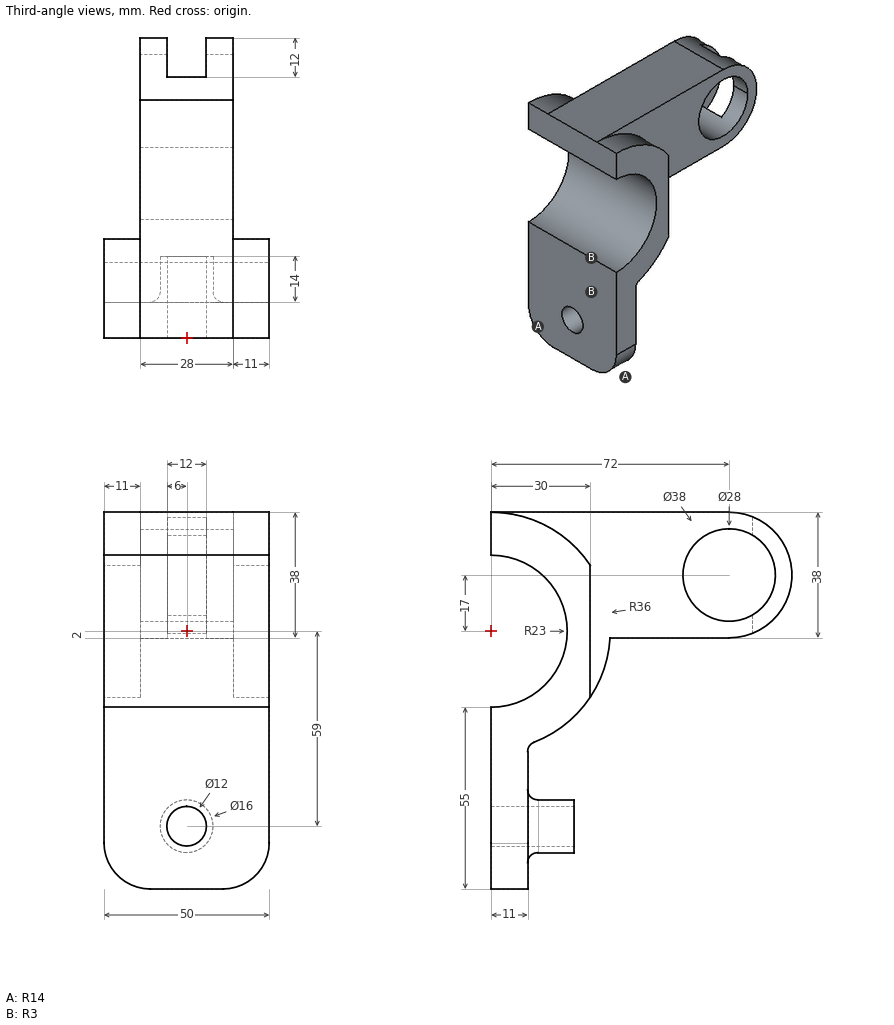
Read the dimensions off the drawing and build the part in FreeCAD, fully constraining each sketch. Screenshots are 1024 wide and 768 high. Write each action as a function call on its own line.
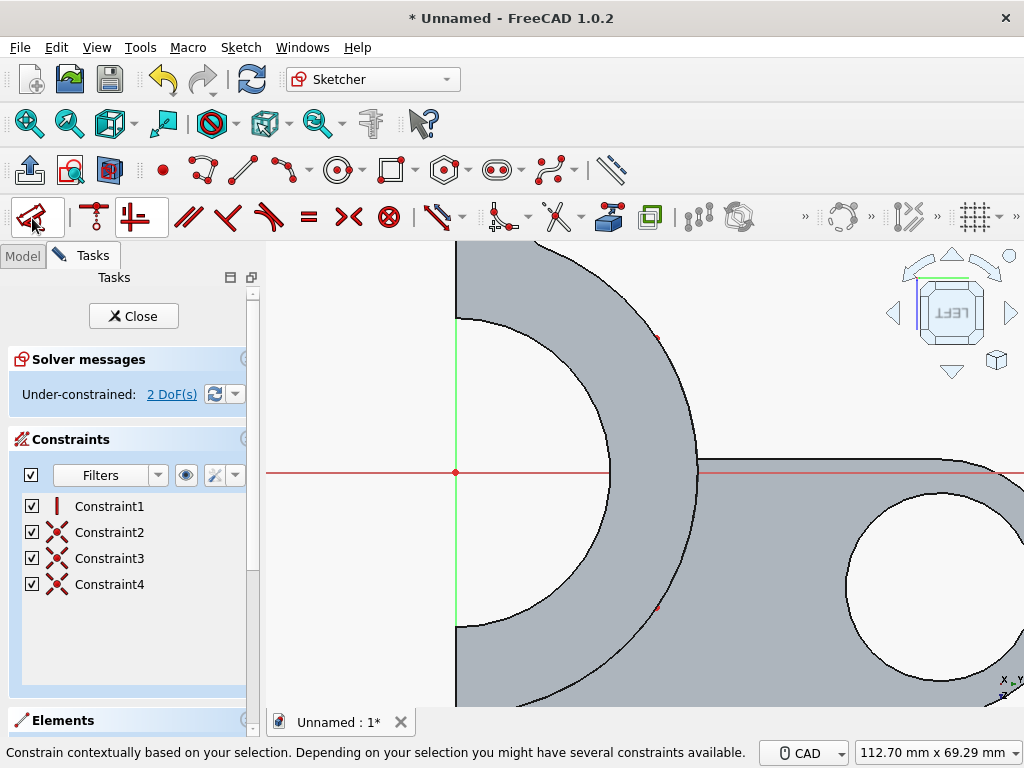
click(691, 529)
click(722, 536)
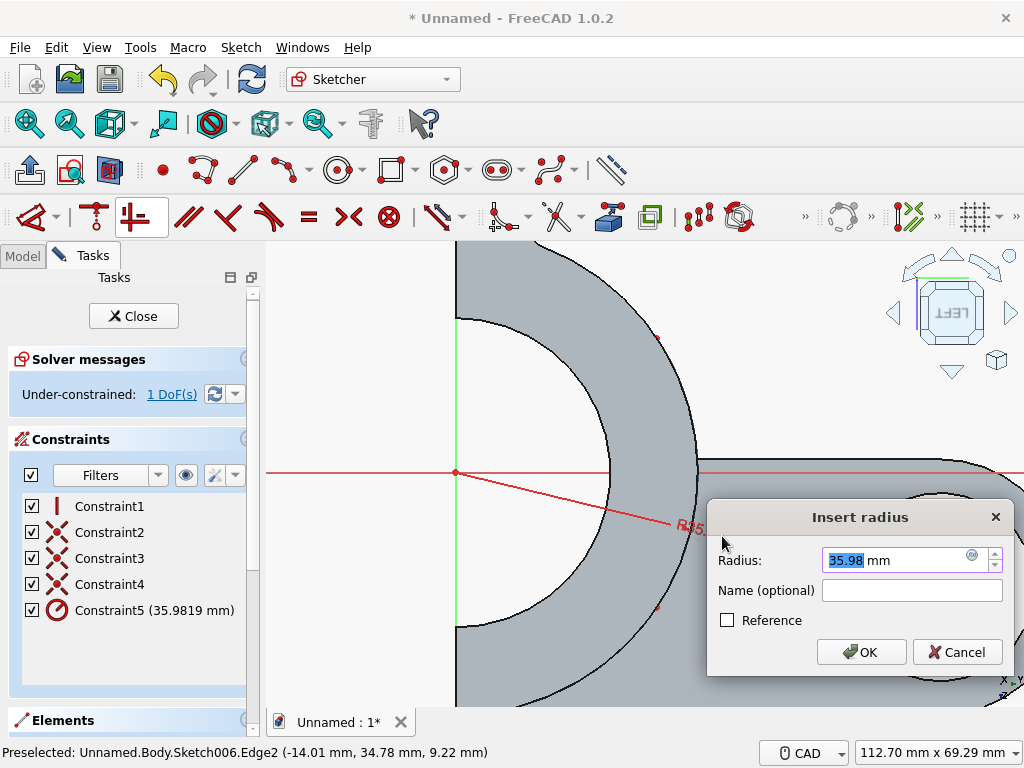
text(36)
key(Return)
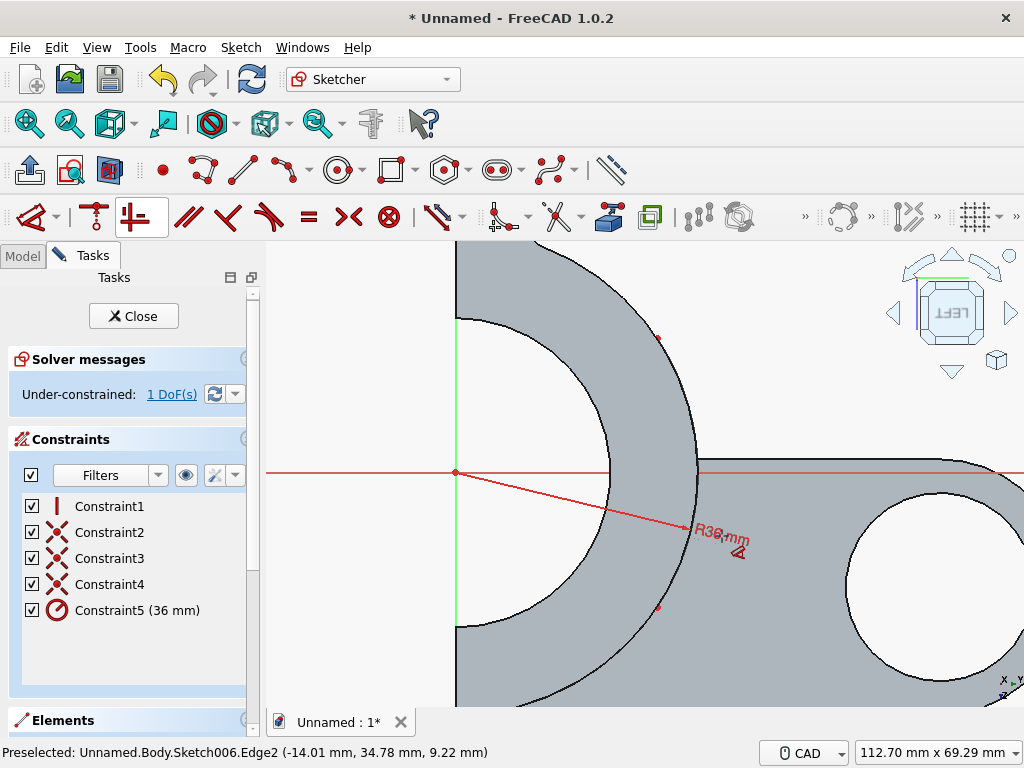
click(657, 338)
click(556, 304)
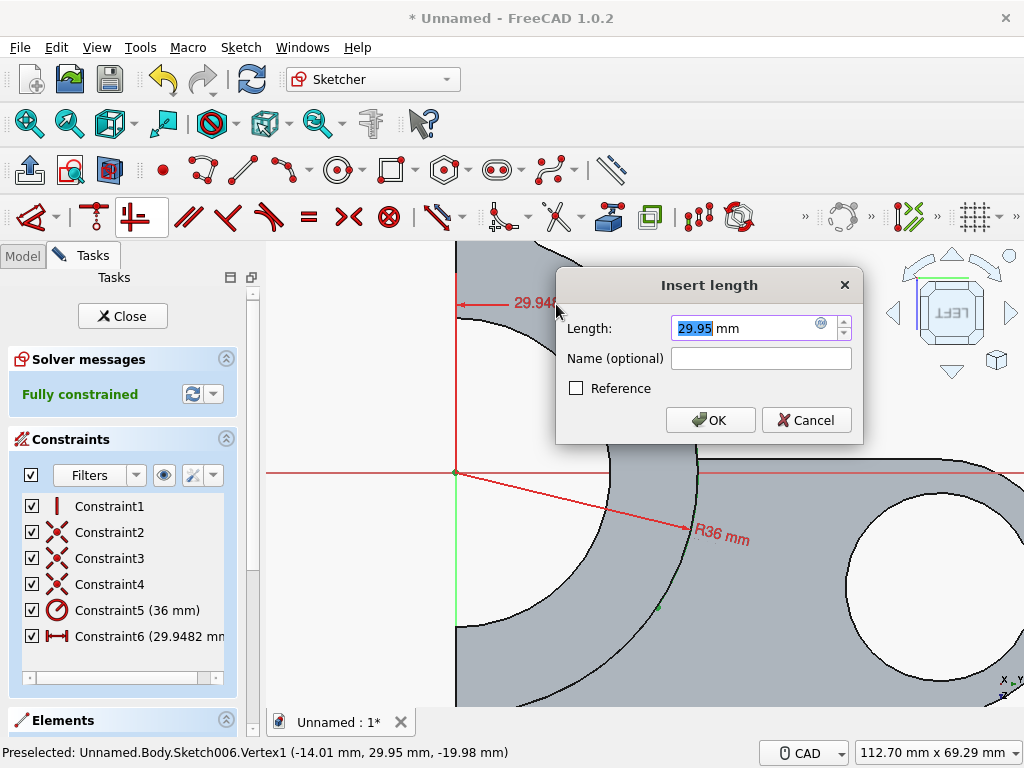
text(30)
key(Return)
key(Escape)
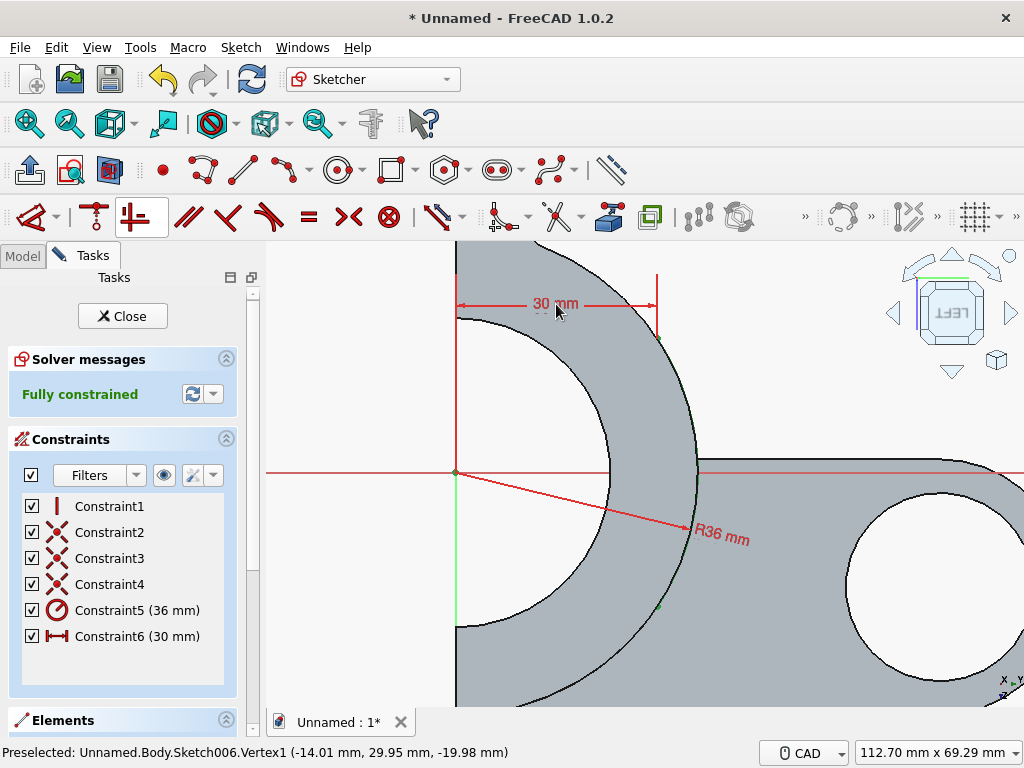
click(123, 316)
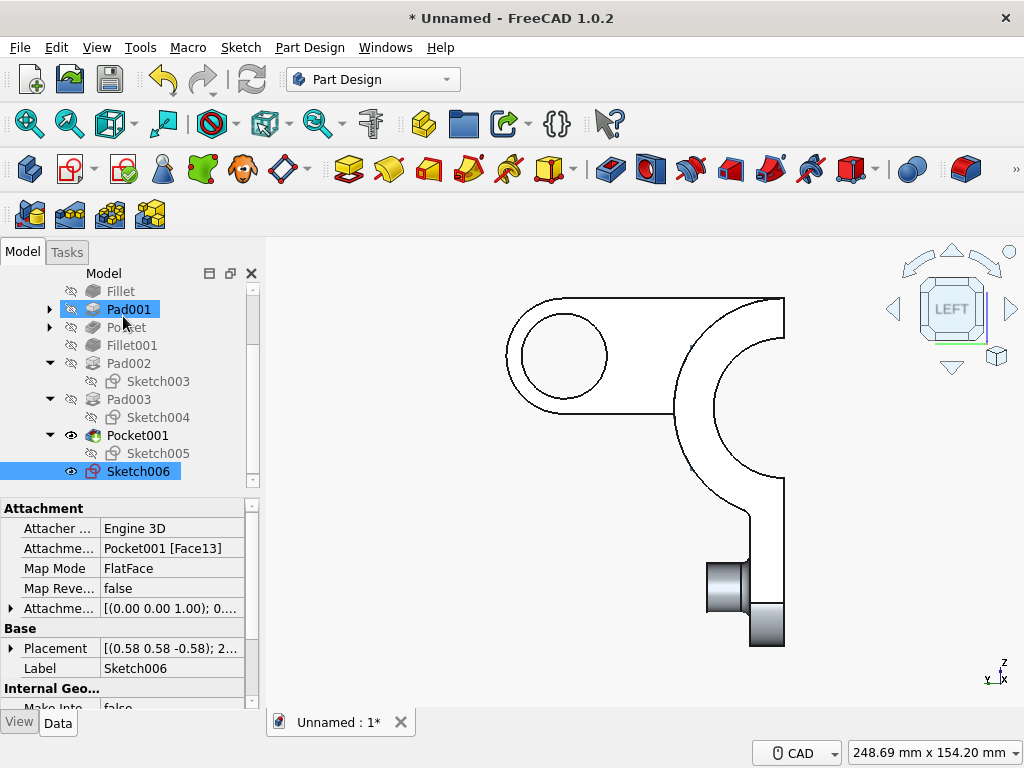
click(612, 170)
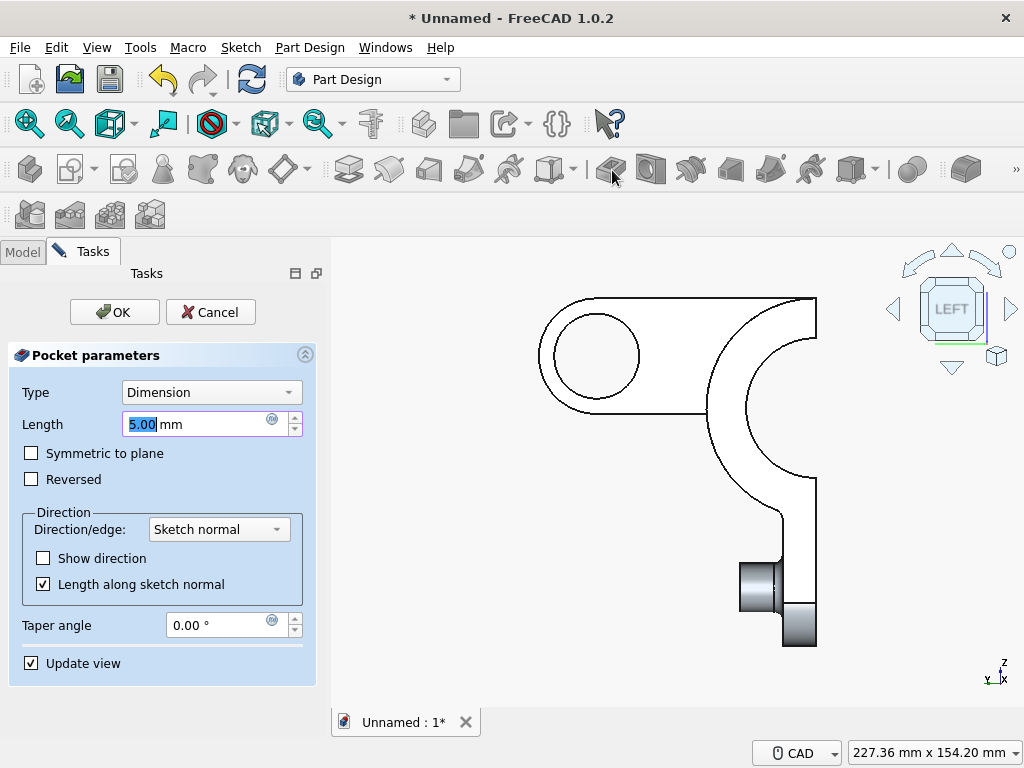
text(11)
key(Tab)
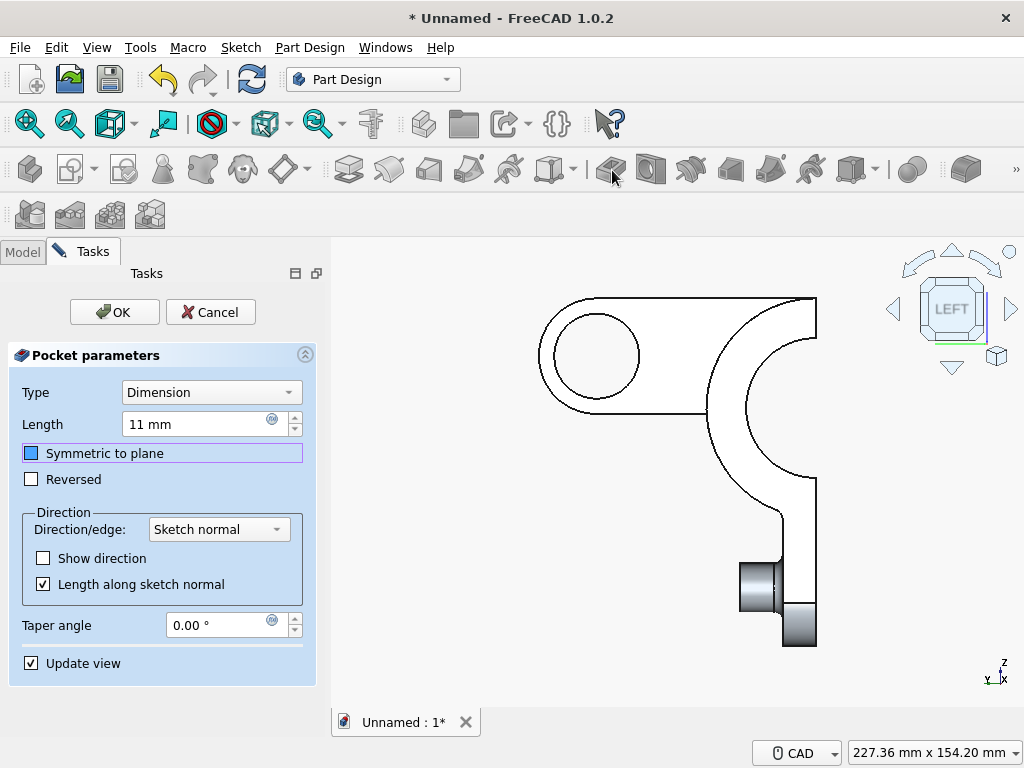
click(30, 479)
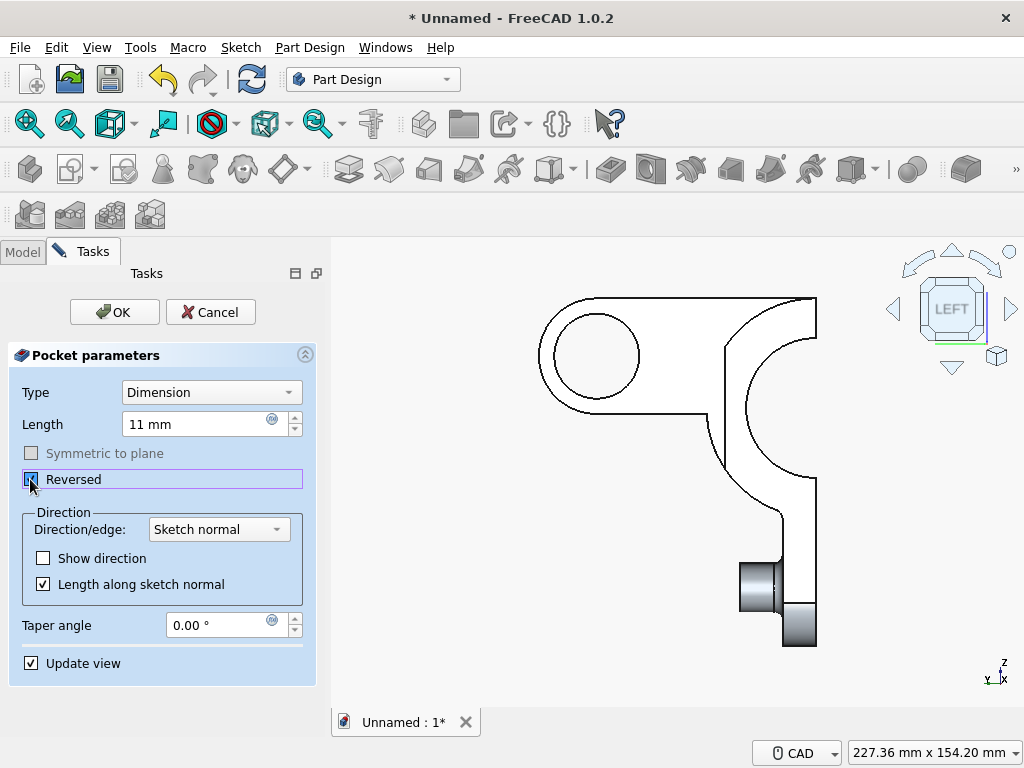
click(115, 312)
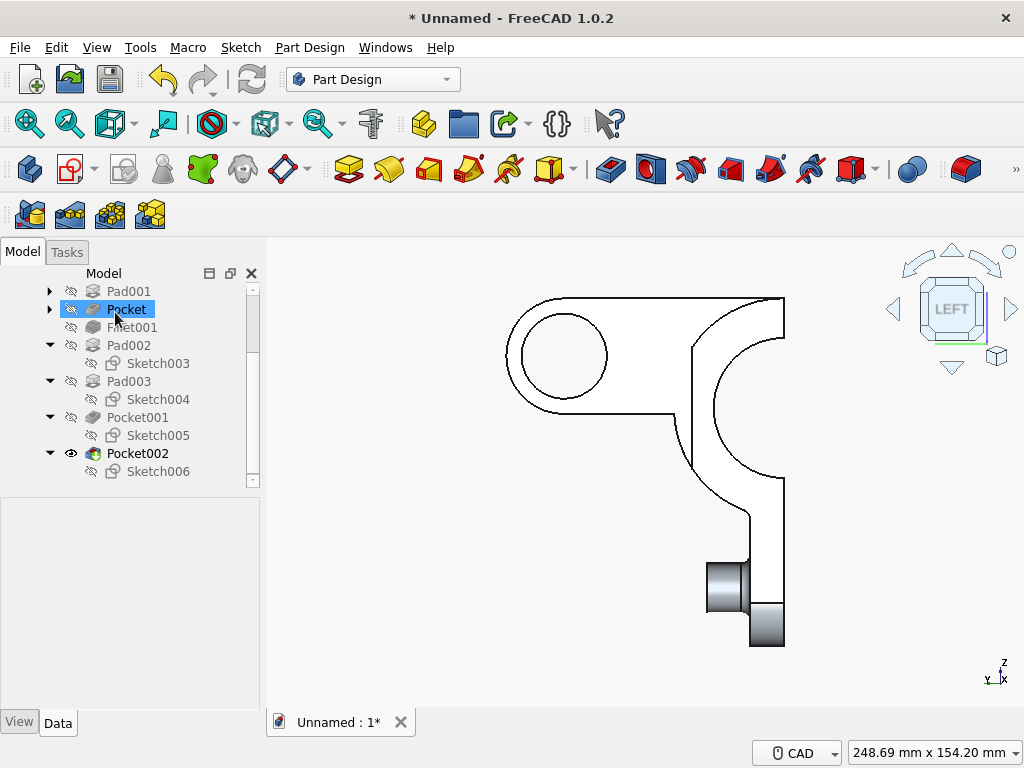
key(0)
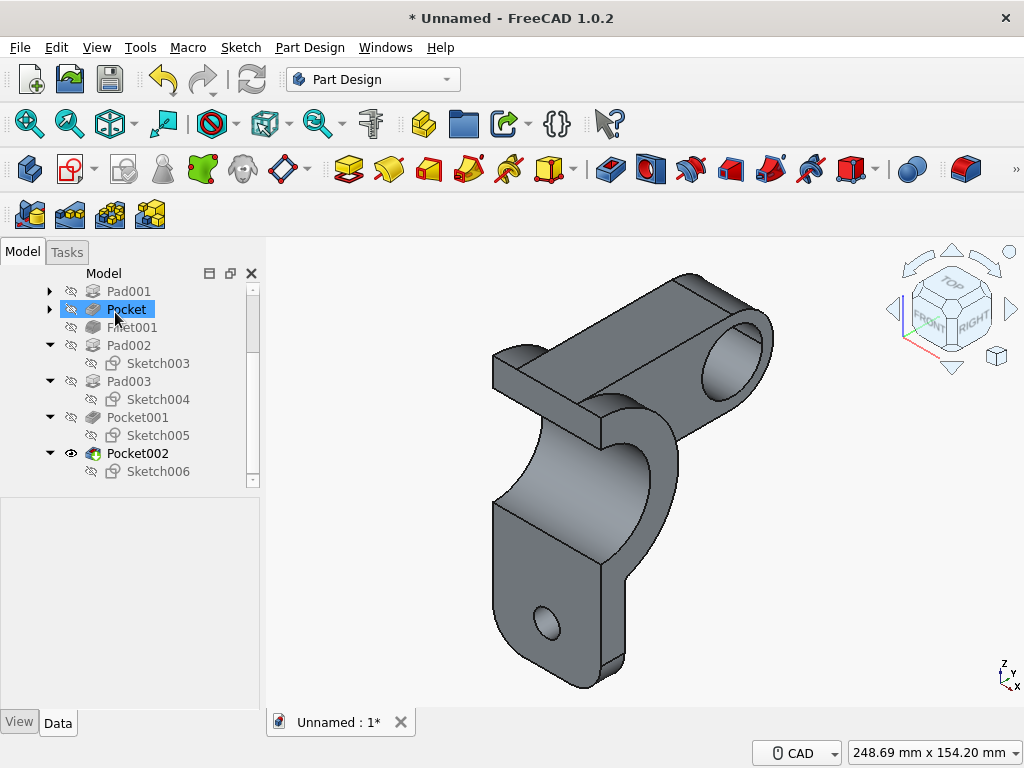
click(617, 567)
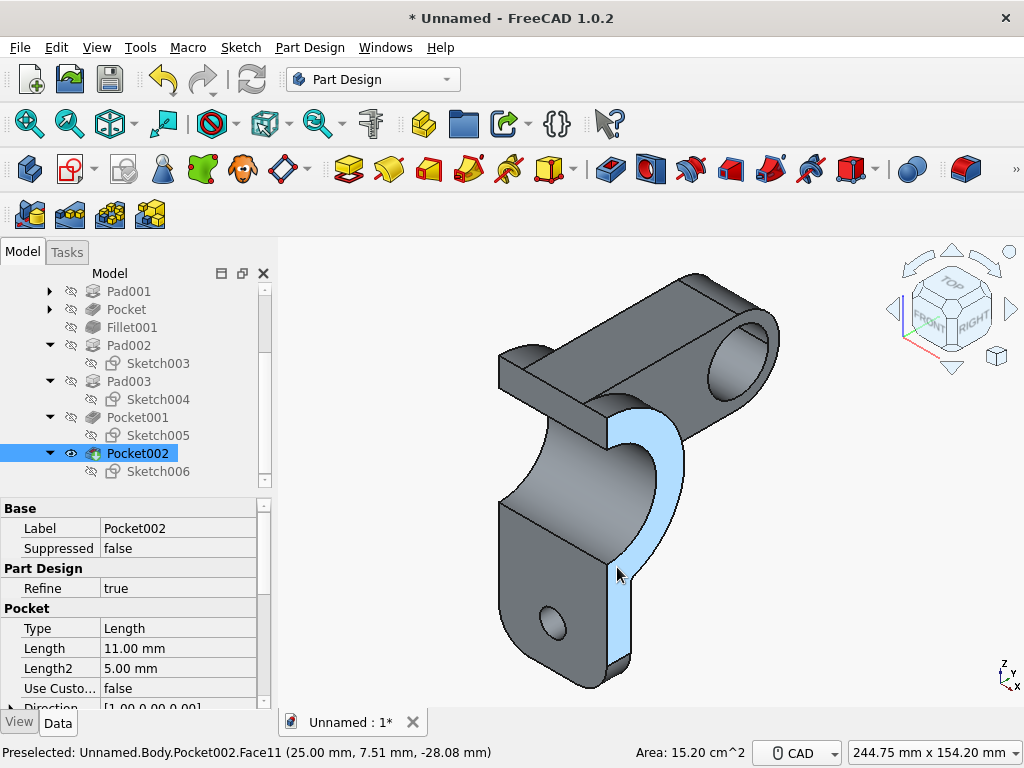
click(70, 170)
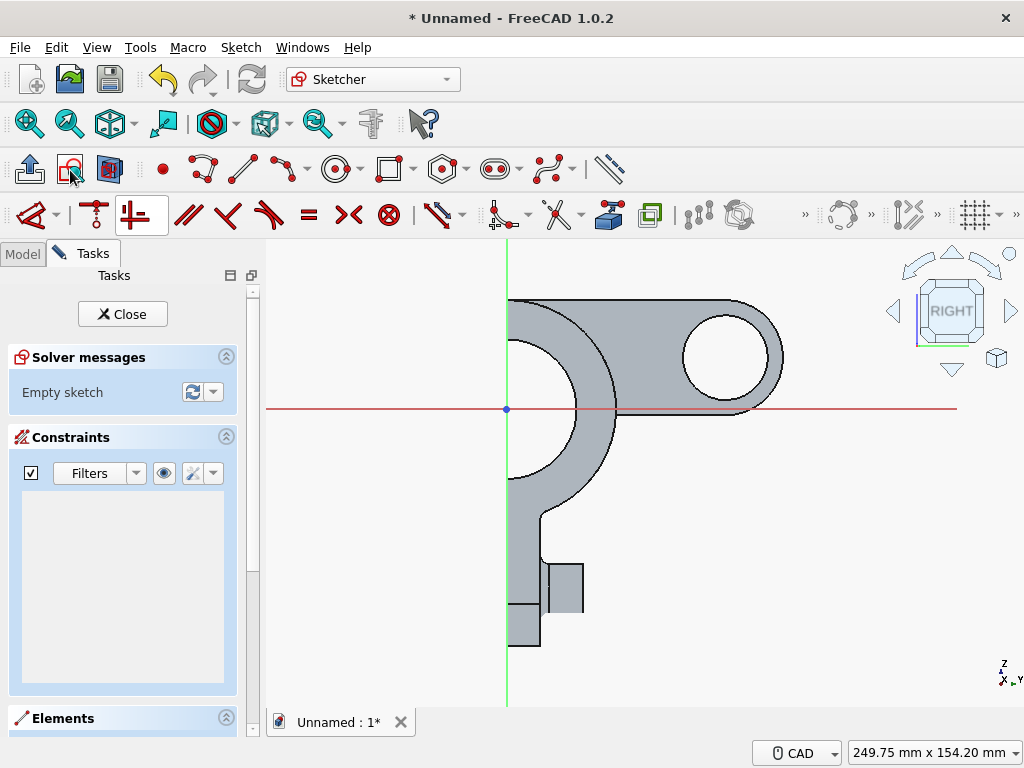
scroll(549, 357, up, 4)